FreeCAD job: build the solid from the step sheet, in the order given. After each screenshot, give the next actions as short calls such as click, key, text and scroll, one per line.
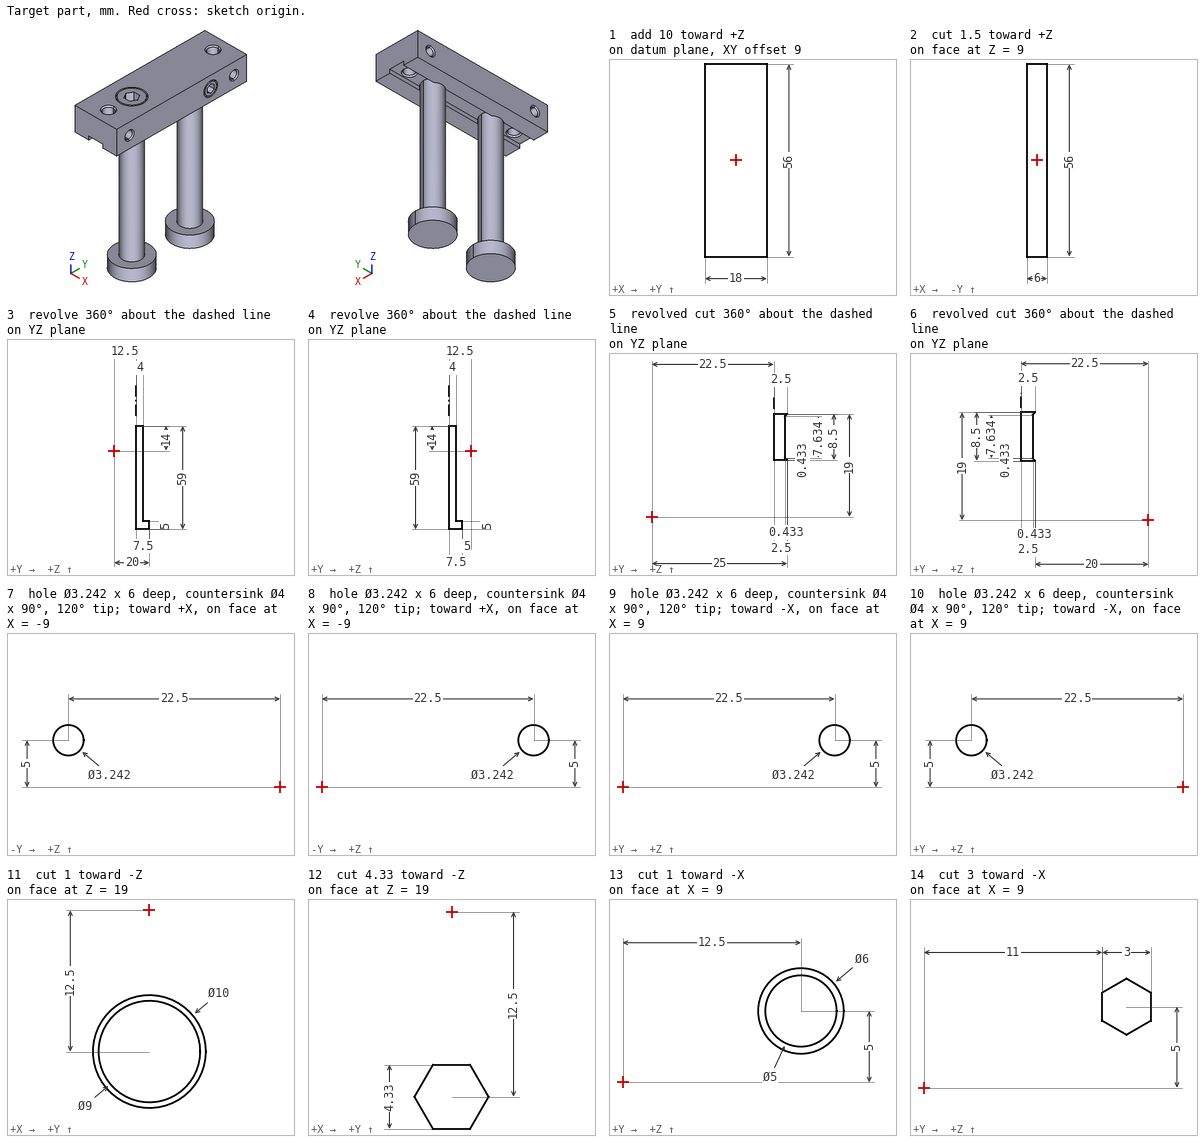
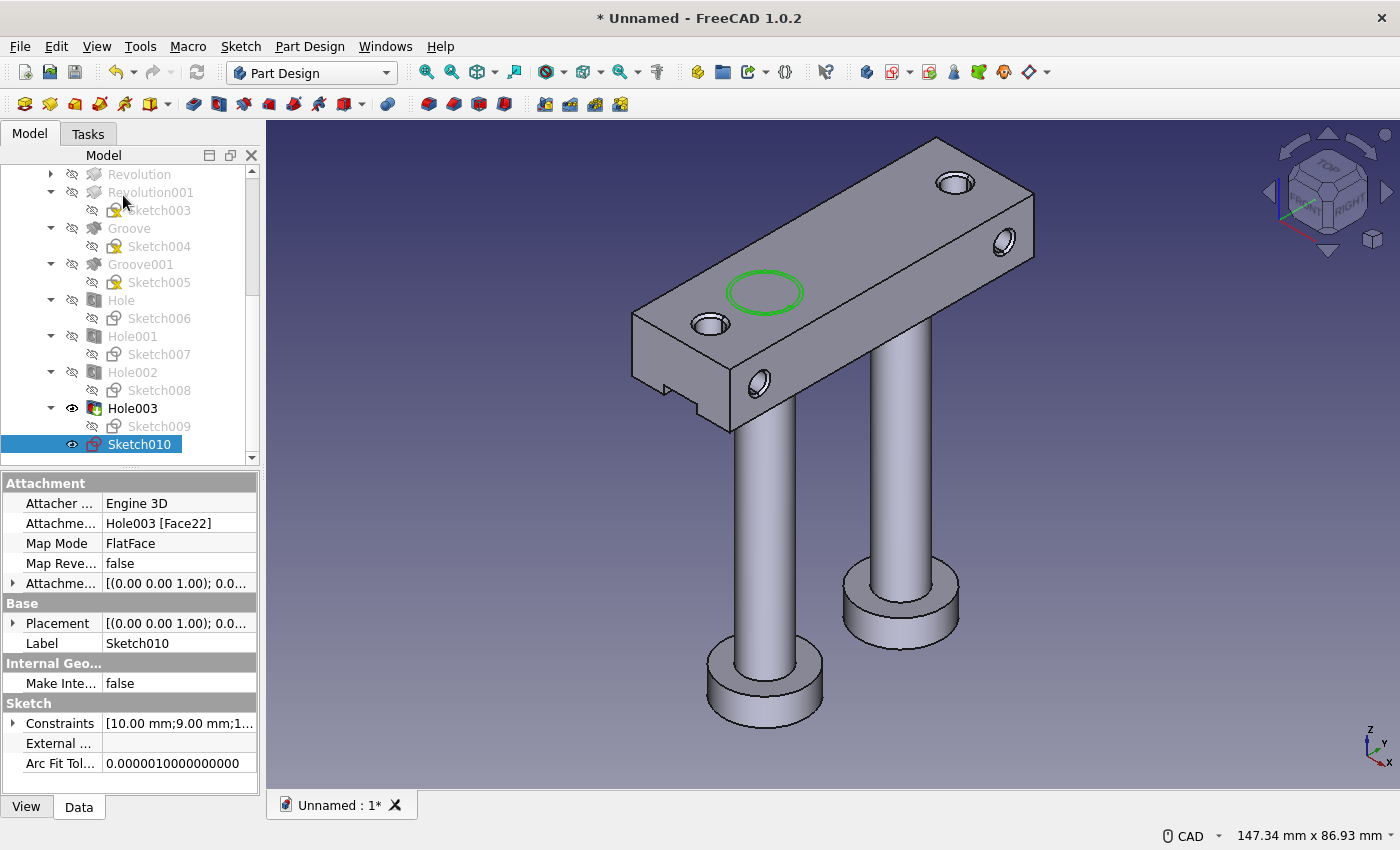
click(194, 104)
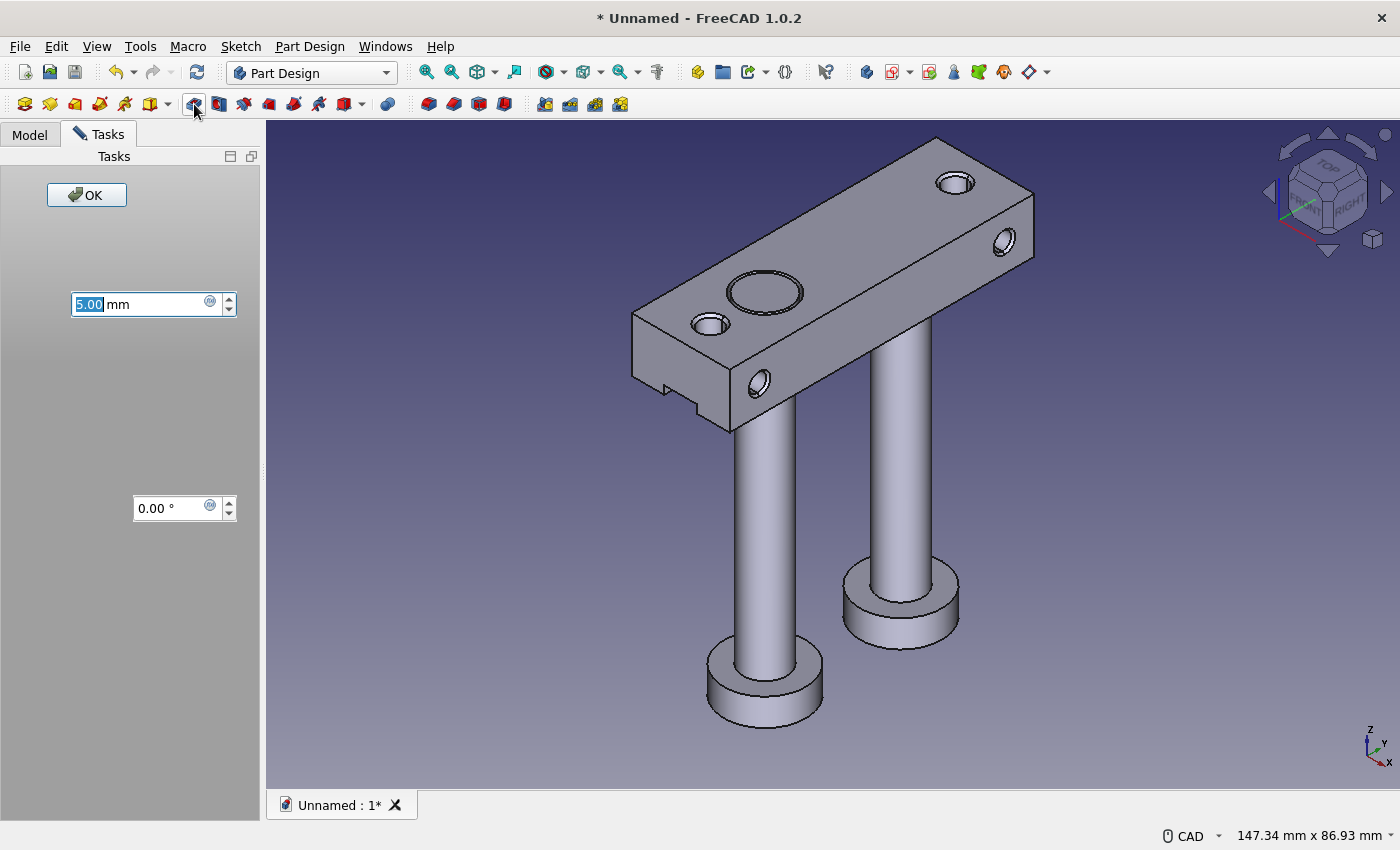
text(1)
key(Tab)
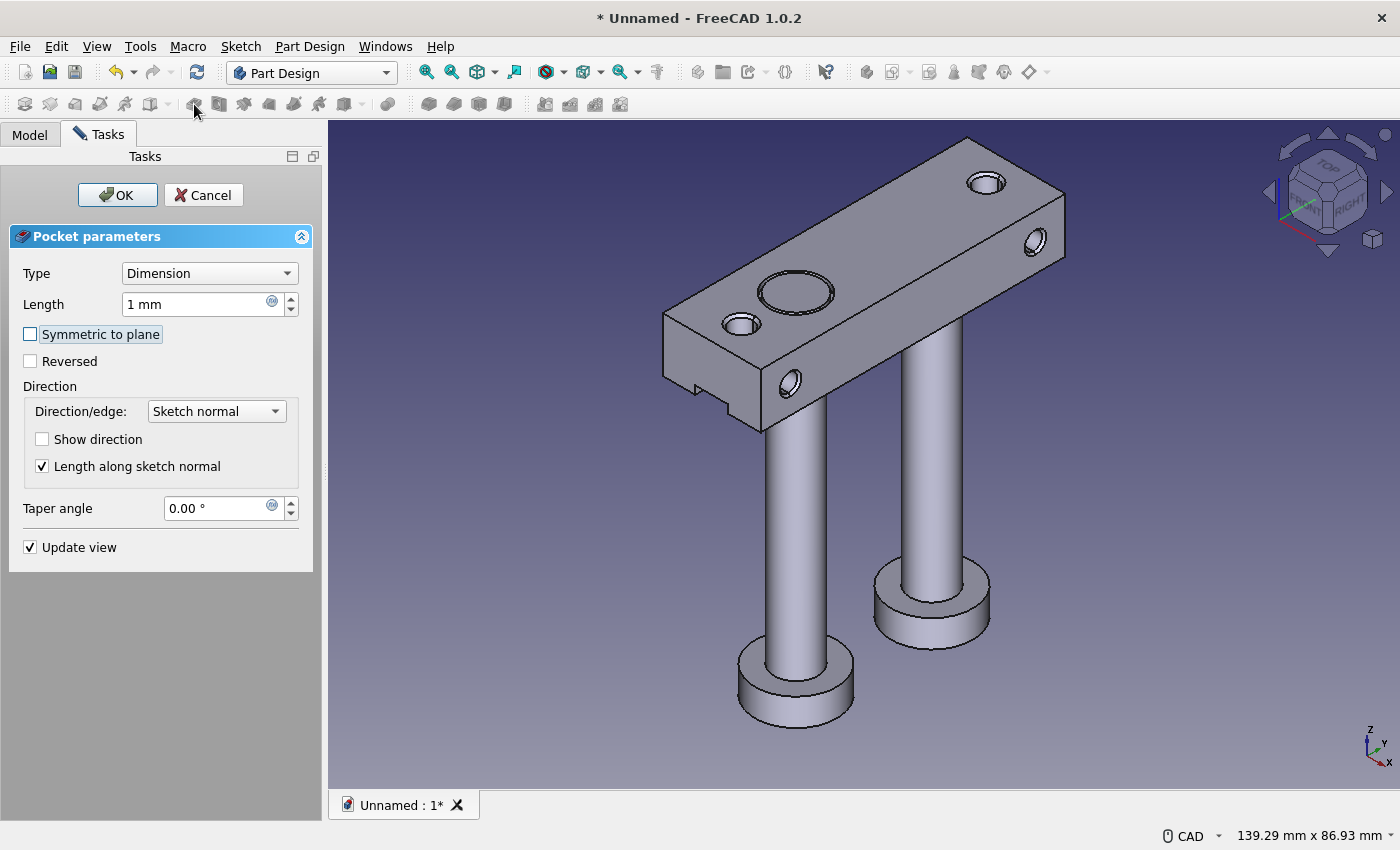
click(118, 195)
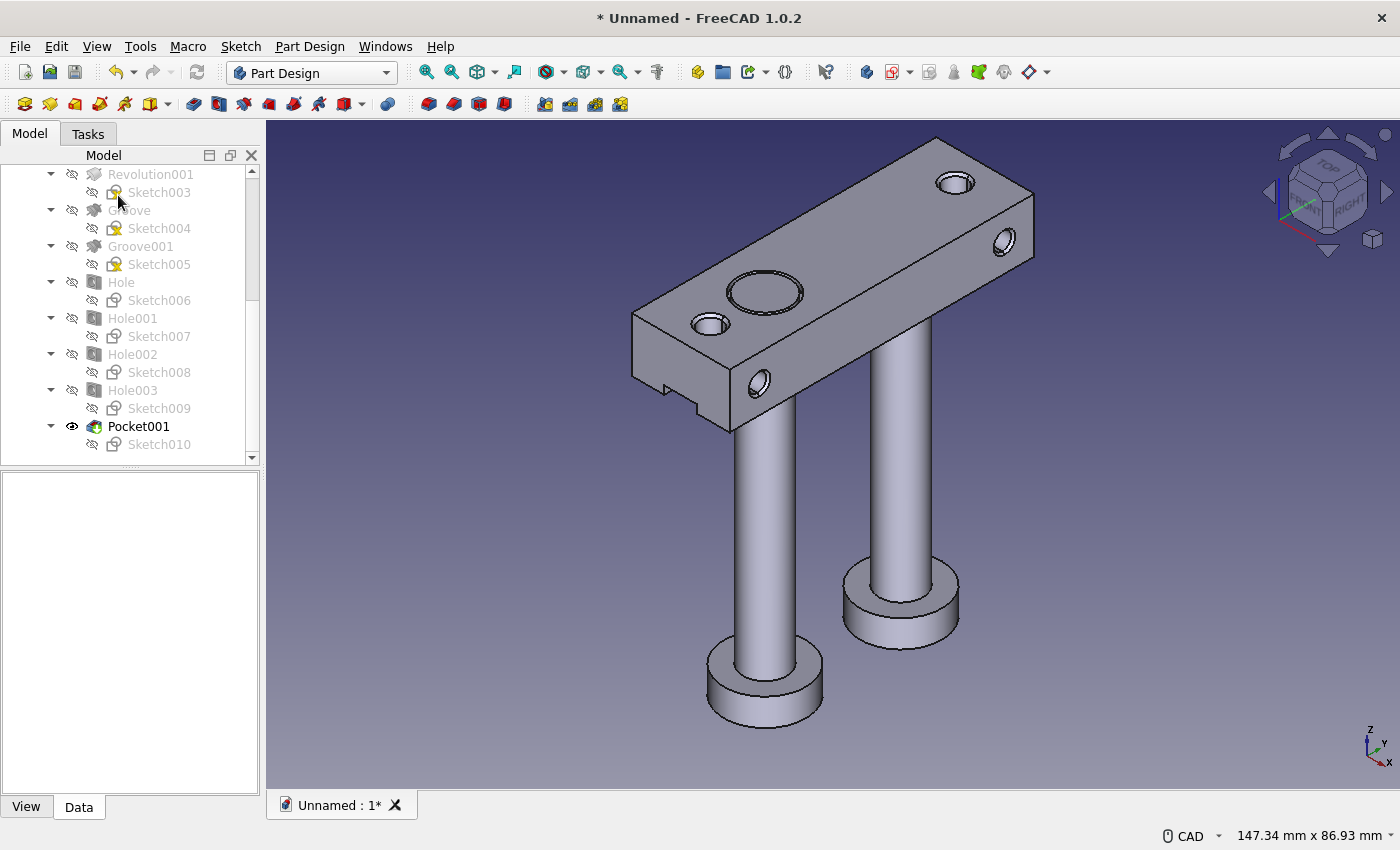
click(877, 227)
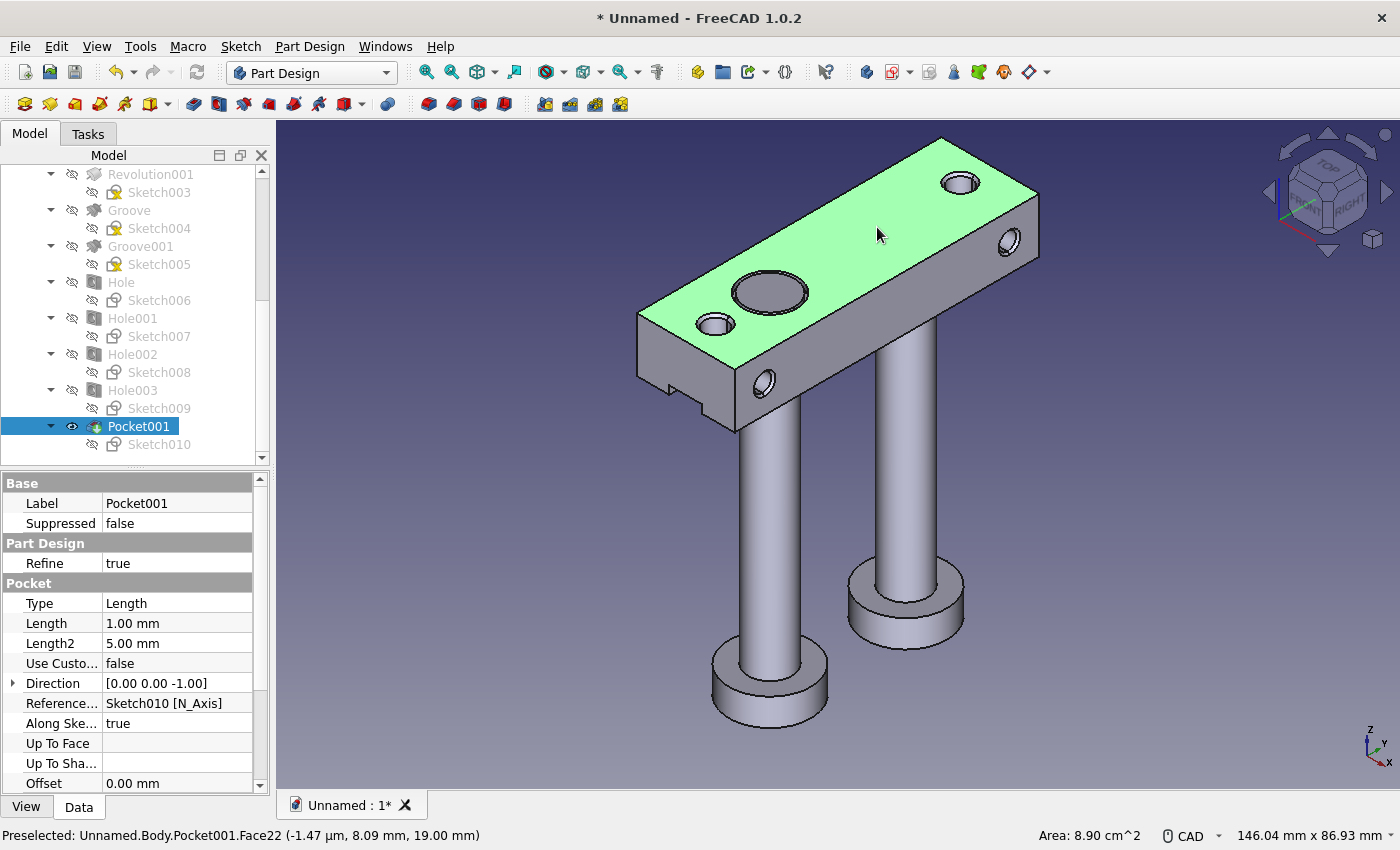
click(892, 72)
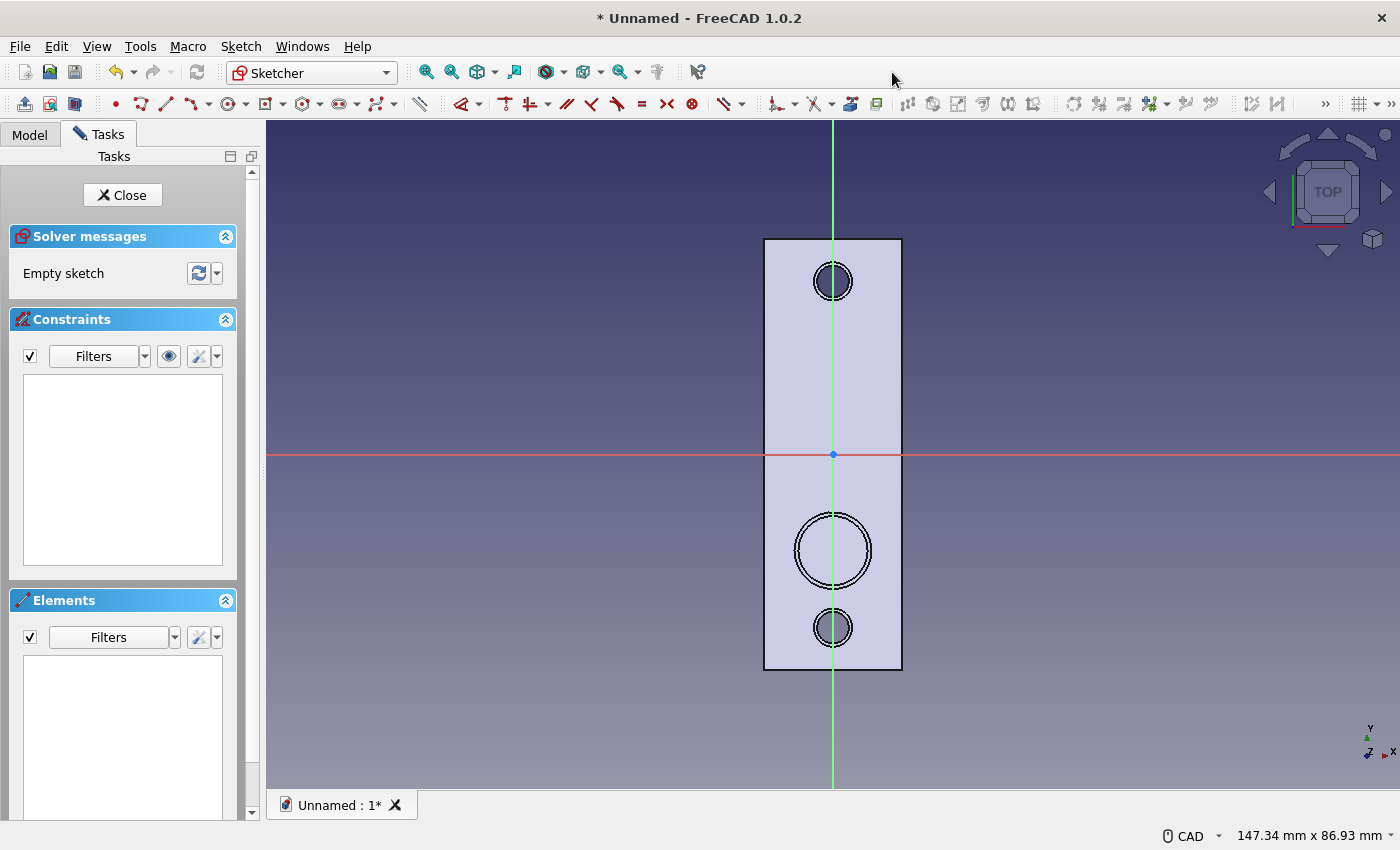
scroll(838, 558, up, 13)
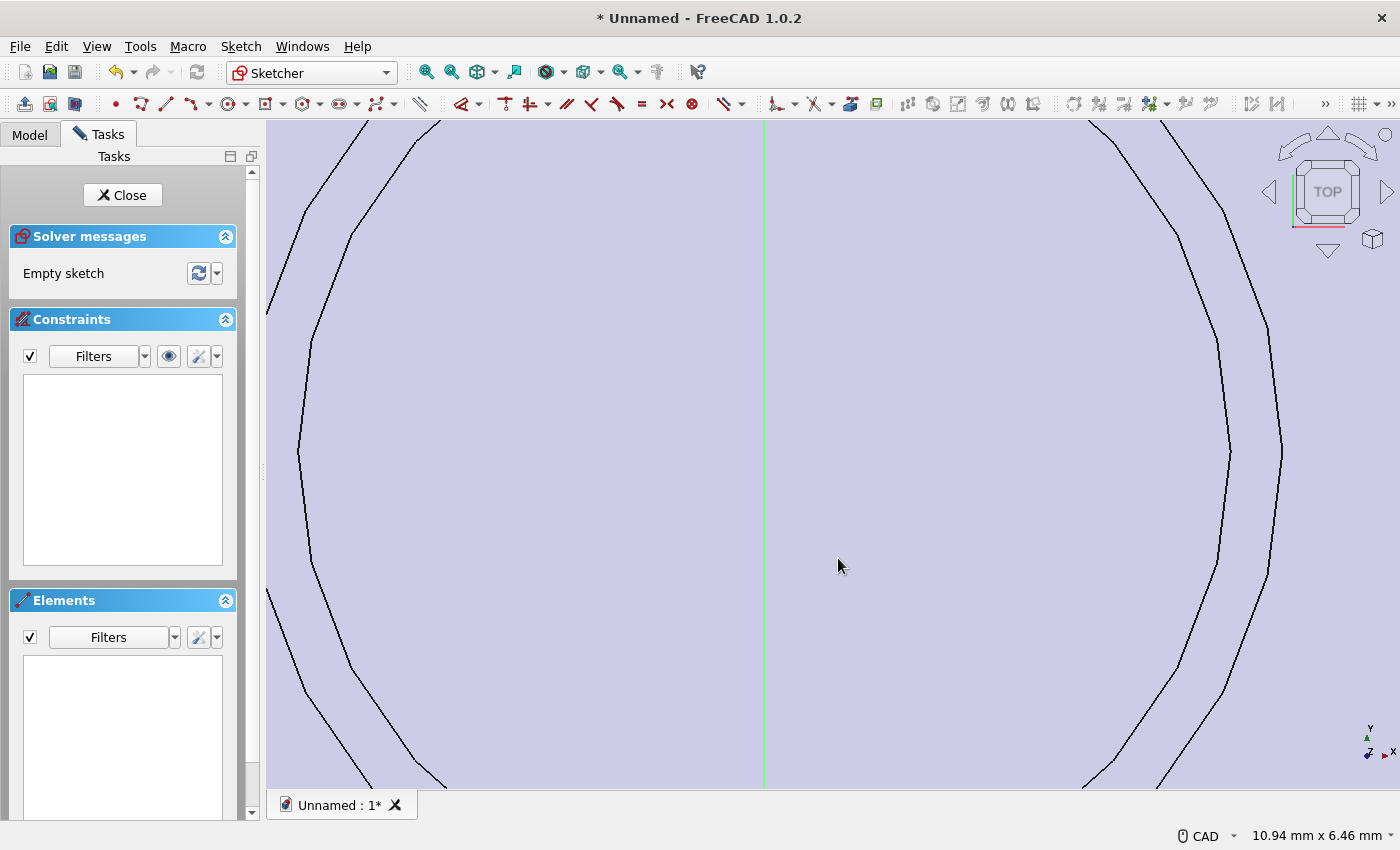
click(302, 104)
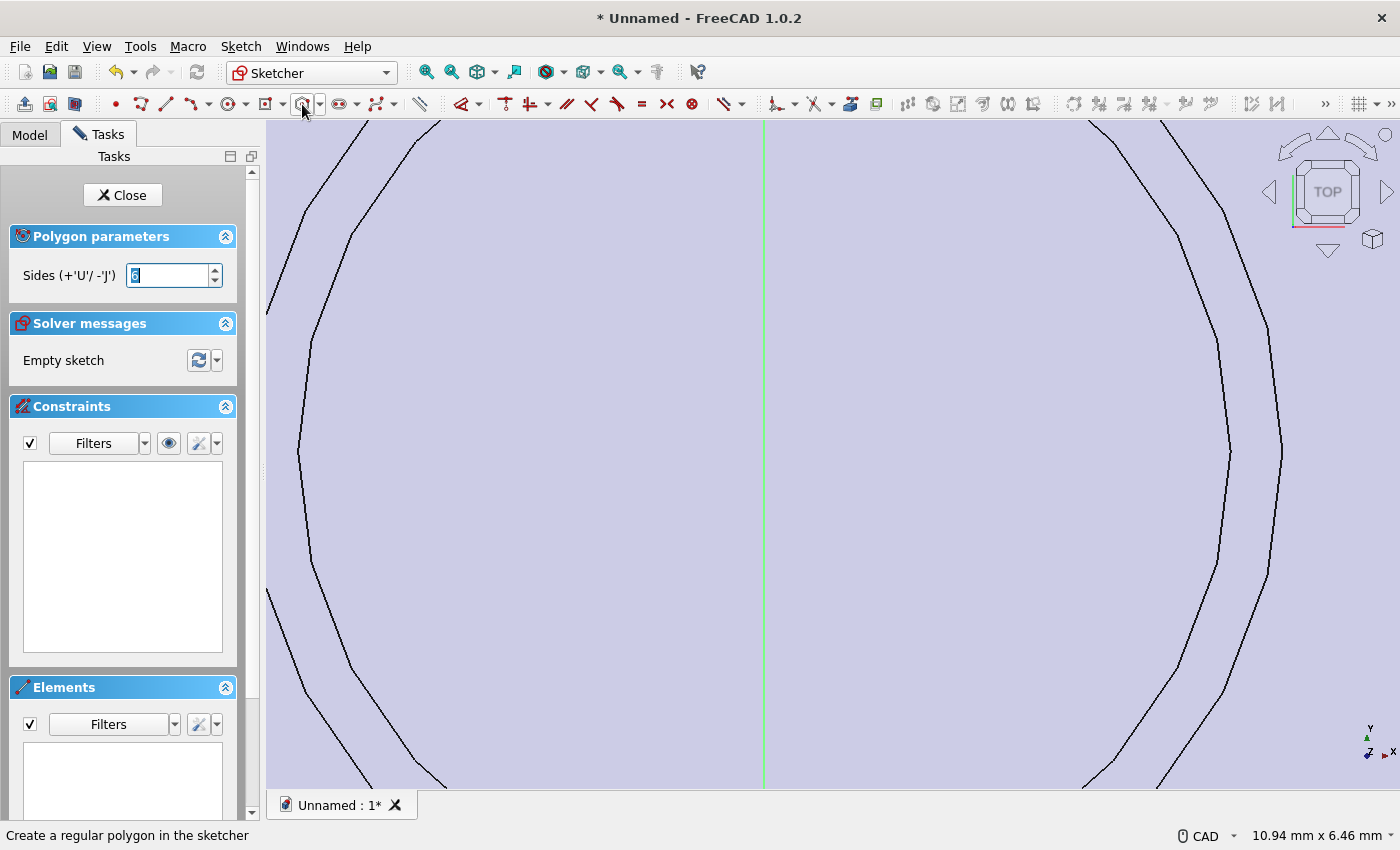
click(764, 452)